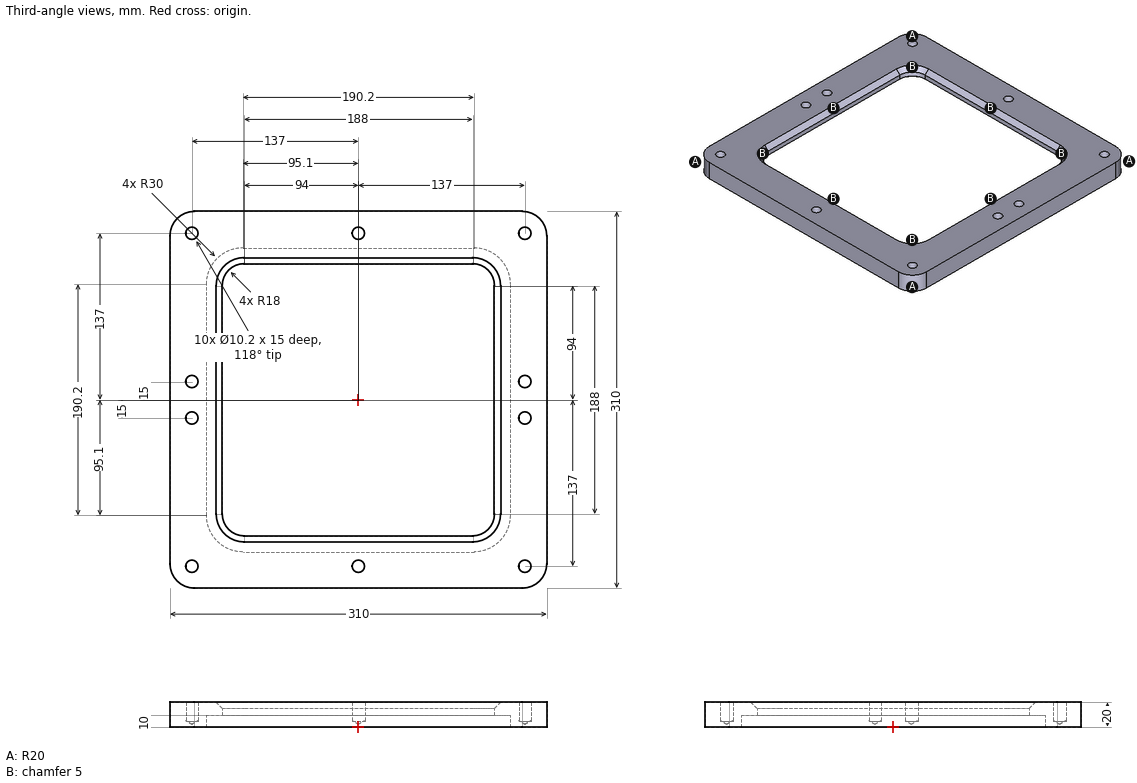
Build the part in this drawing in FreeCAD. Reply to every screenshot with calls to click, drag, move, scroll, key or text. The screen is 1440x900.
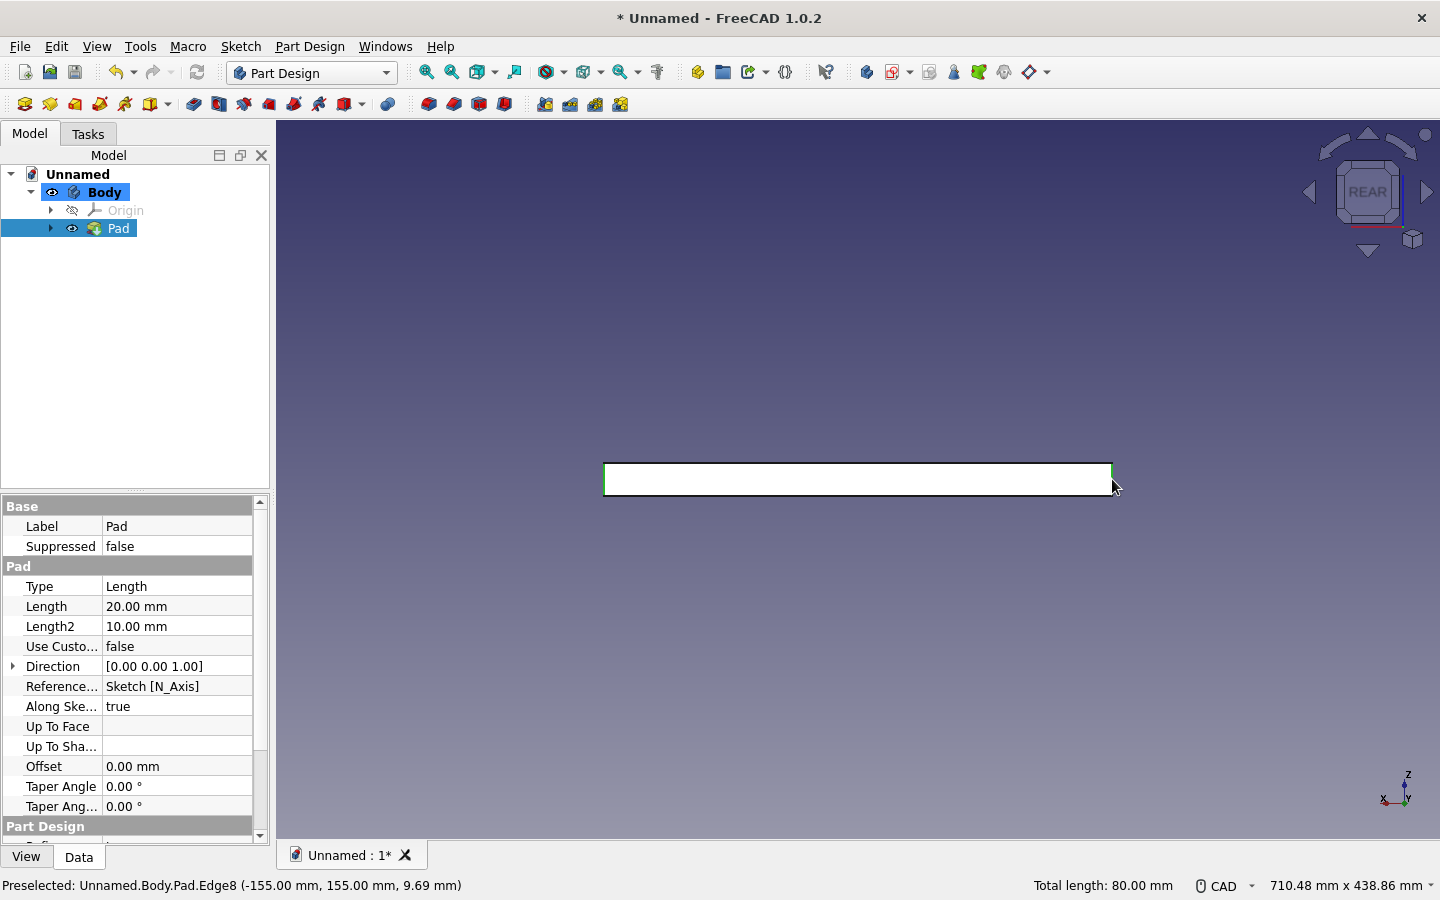
click(429, 104)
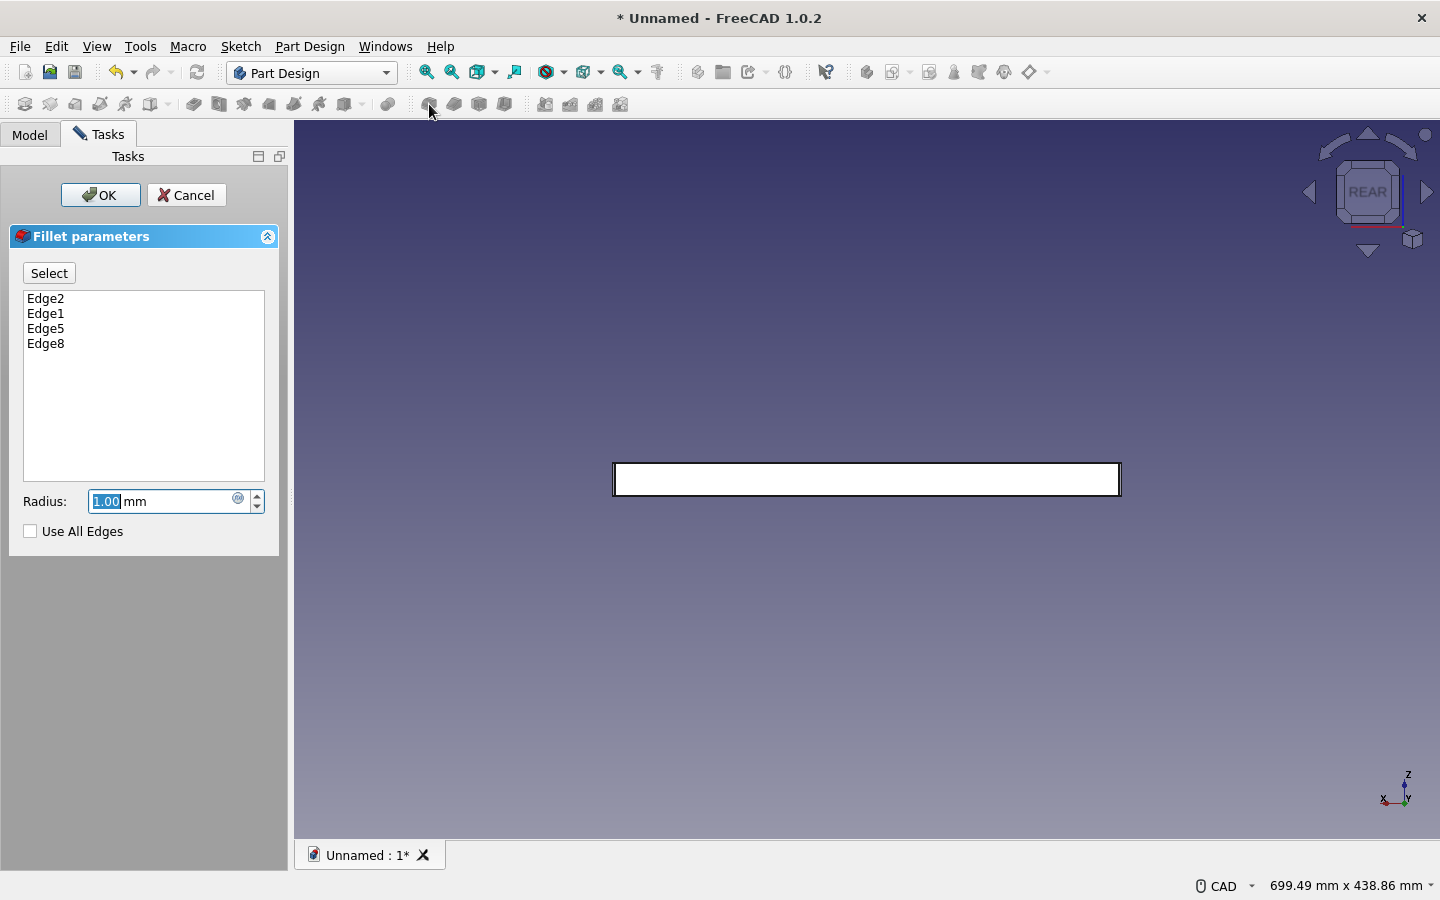
text(20)
key(Tab)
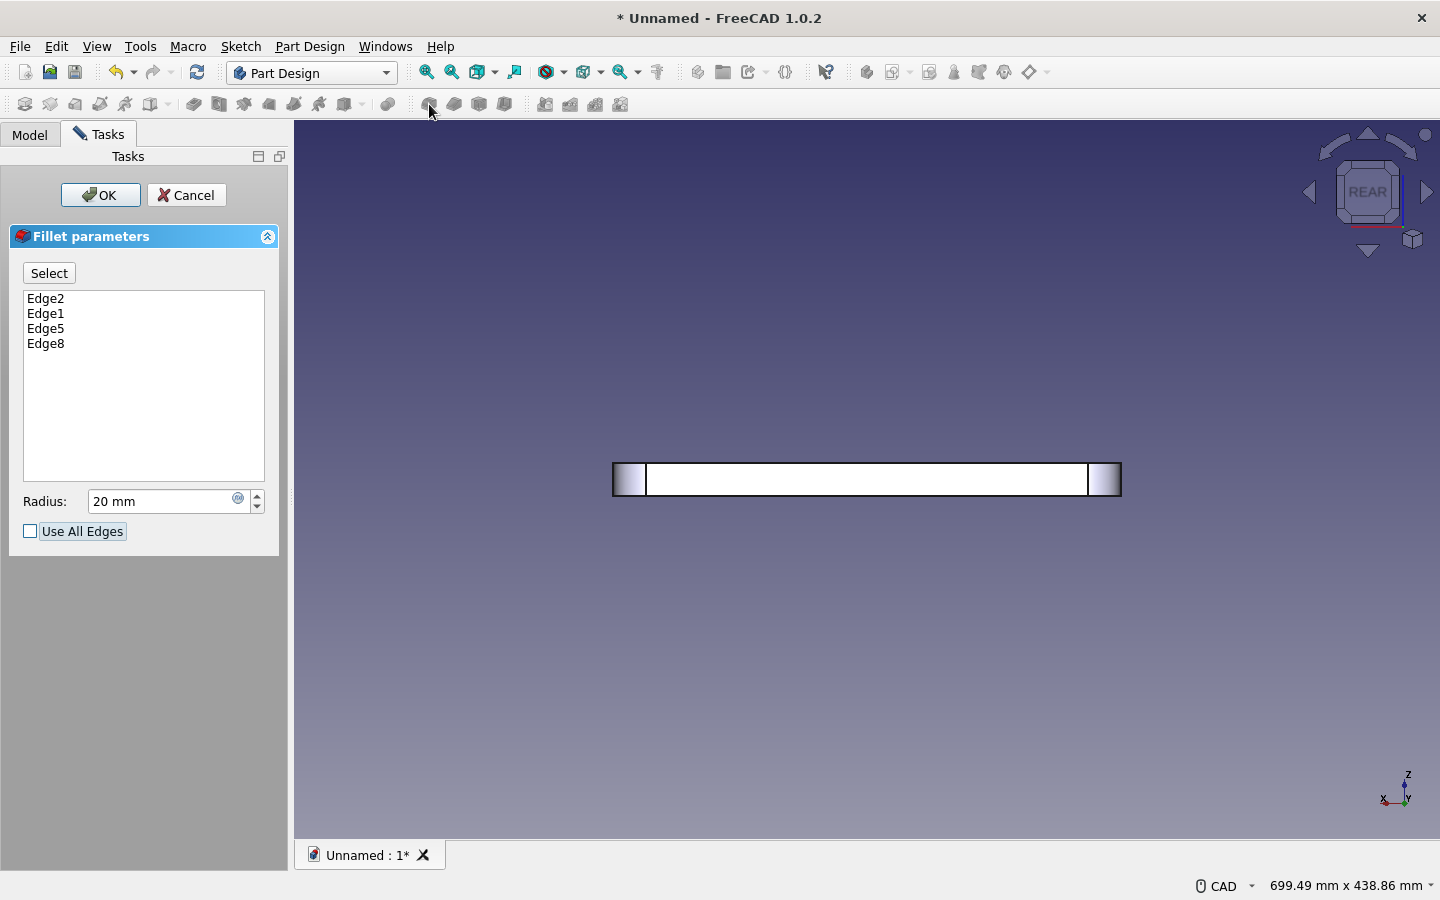
click(101, 195)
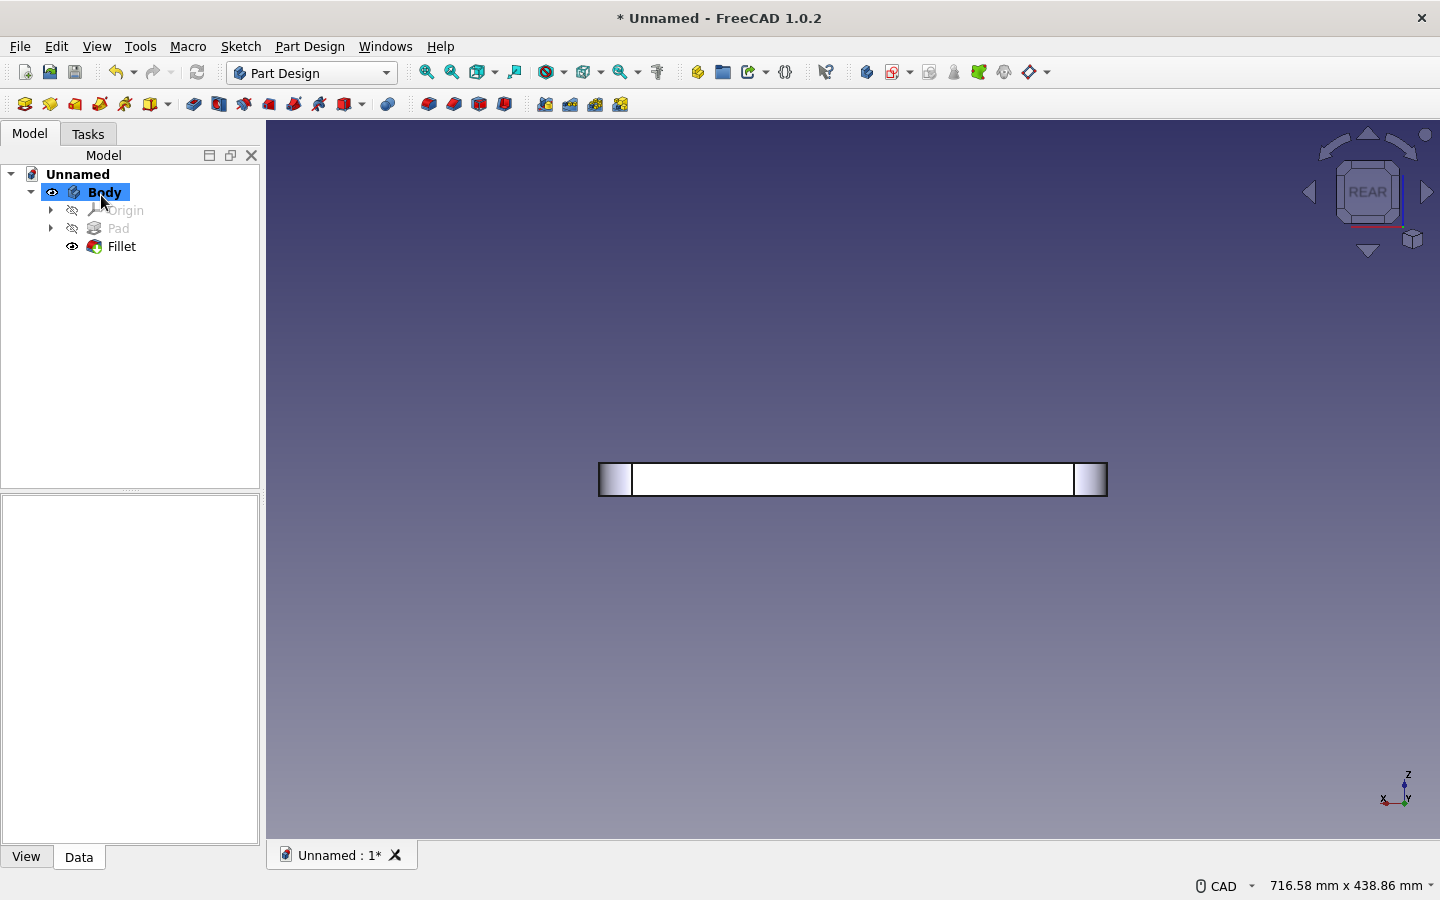
click(427, 72)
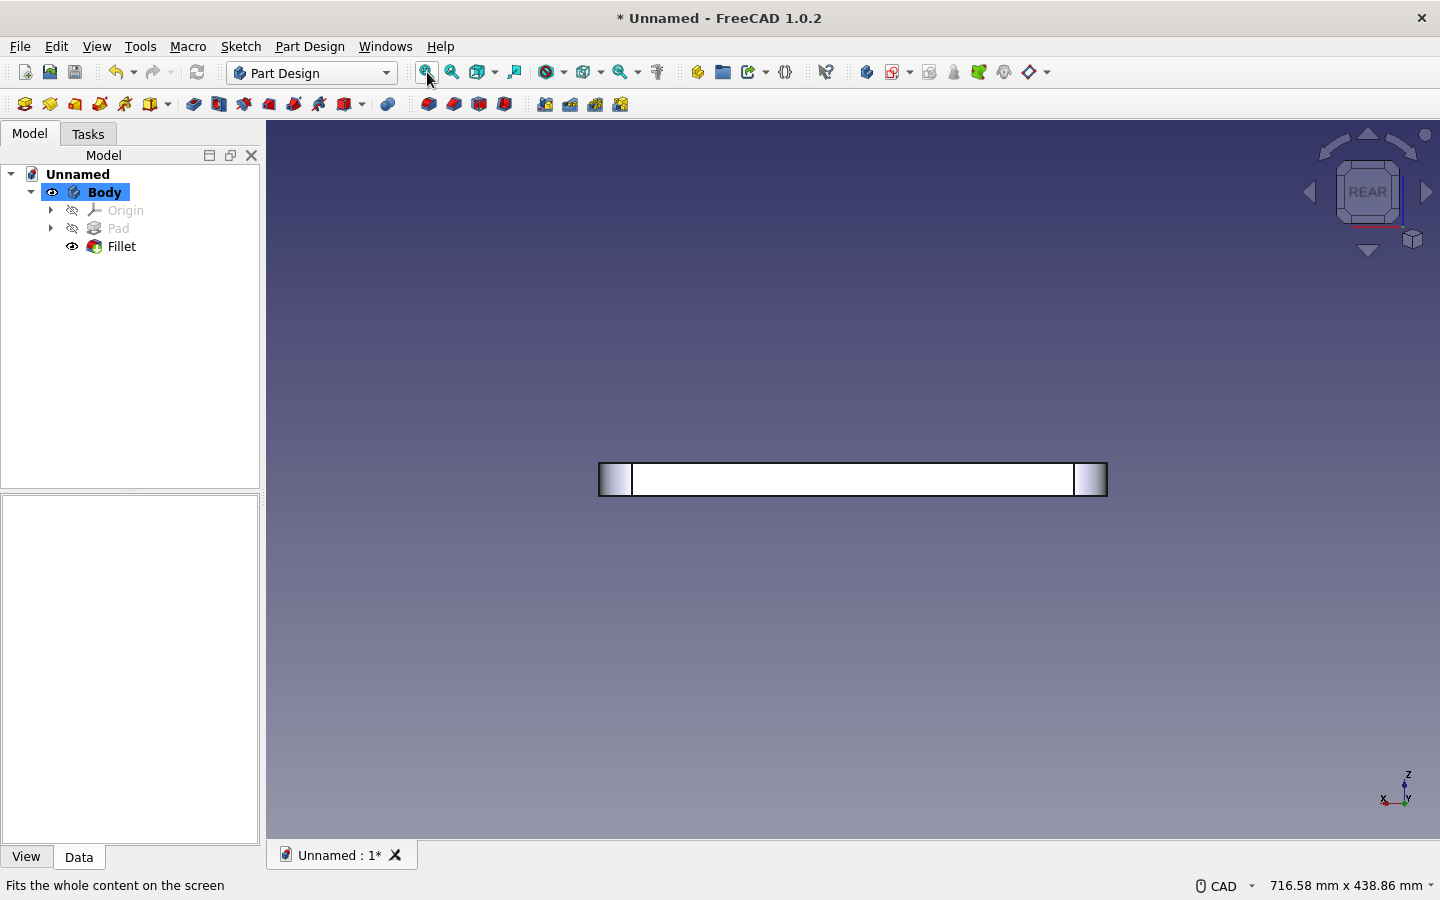
key(5)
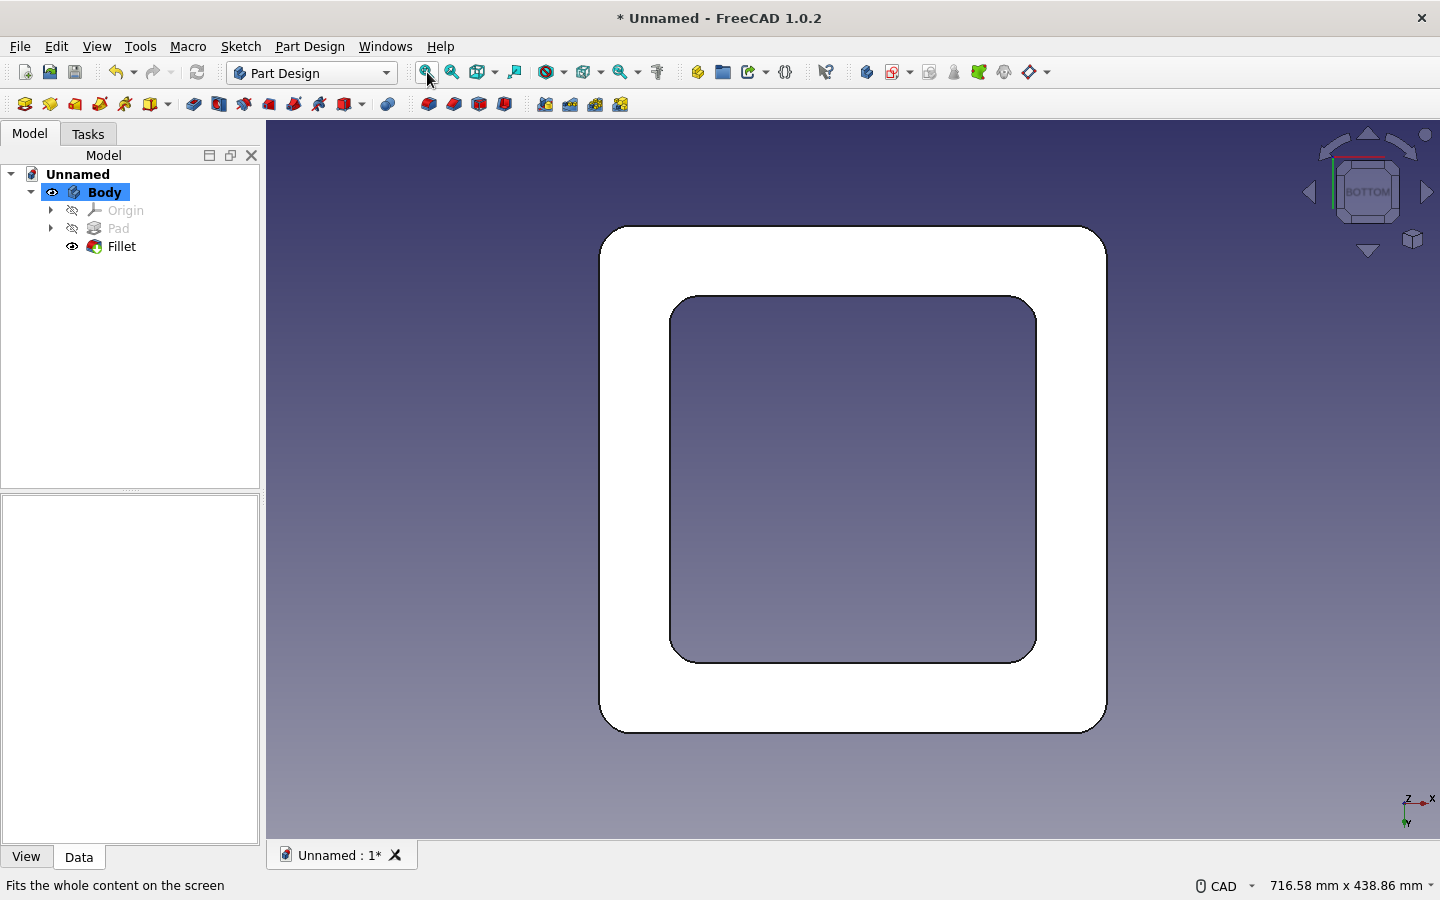
click(1071, 696)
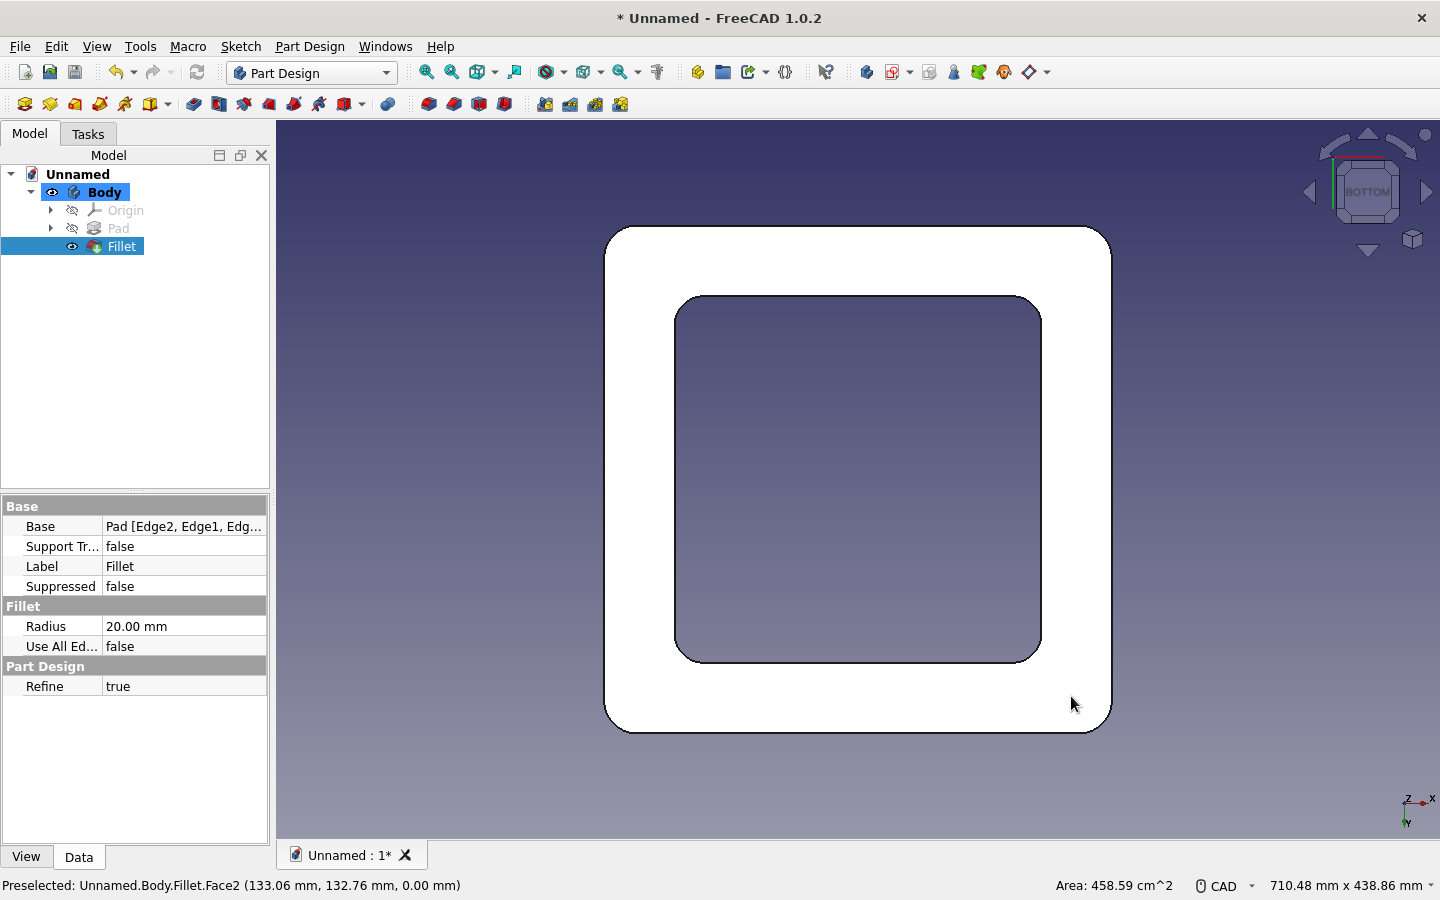
click(892, 72)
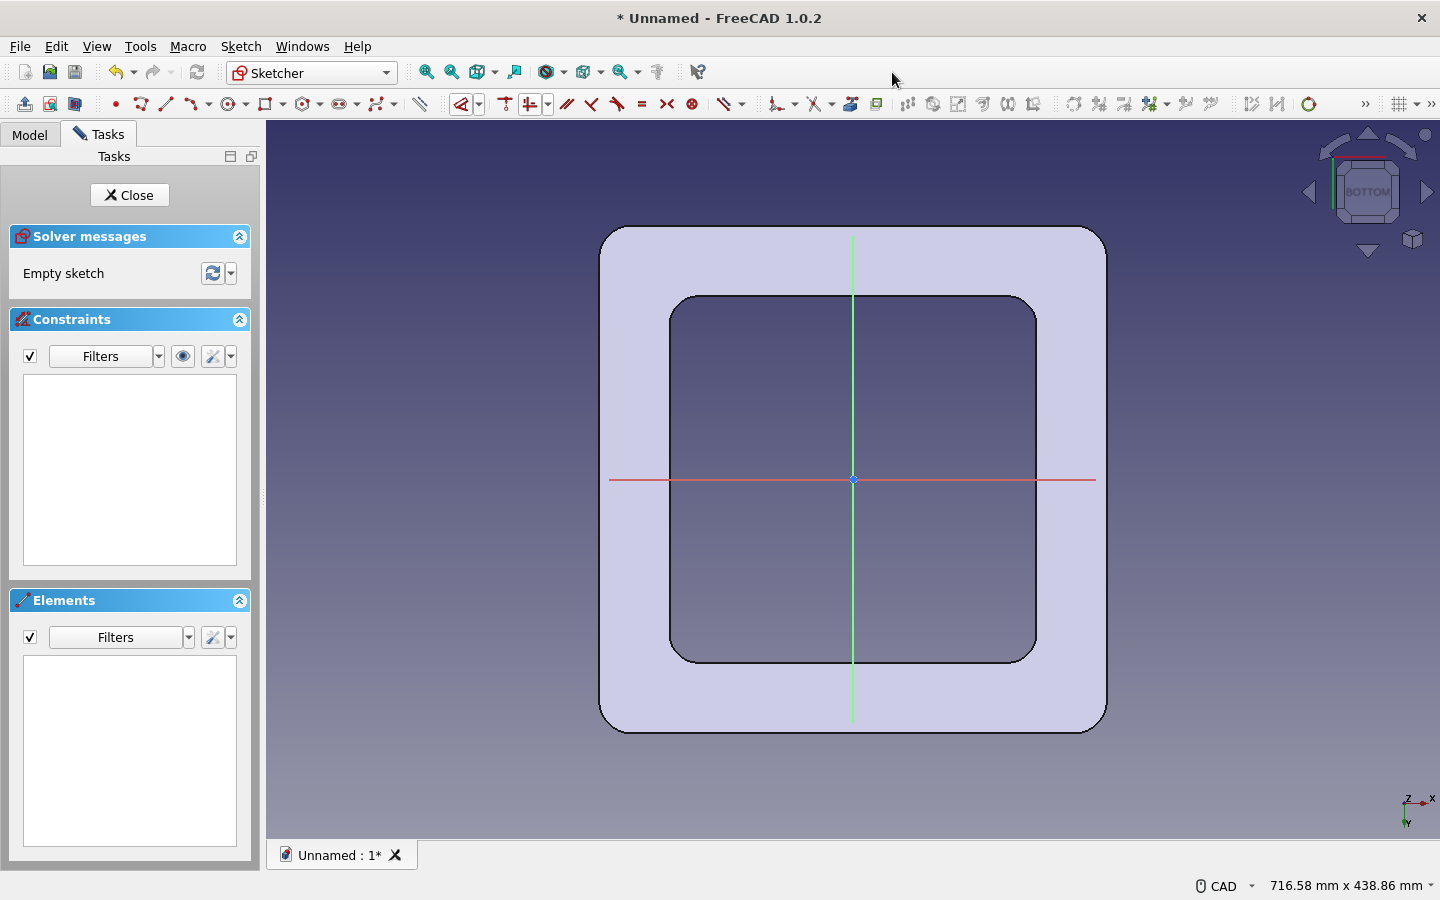
click(166, 104)